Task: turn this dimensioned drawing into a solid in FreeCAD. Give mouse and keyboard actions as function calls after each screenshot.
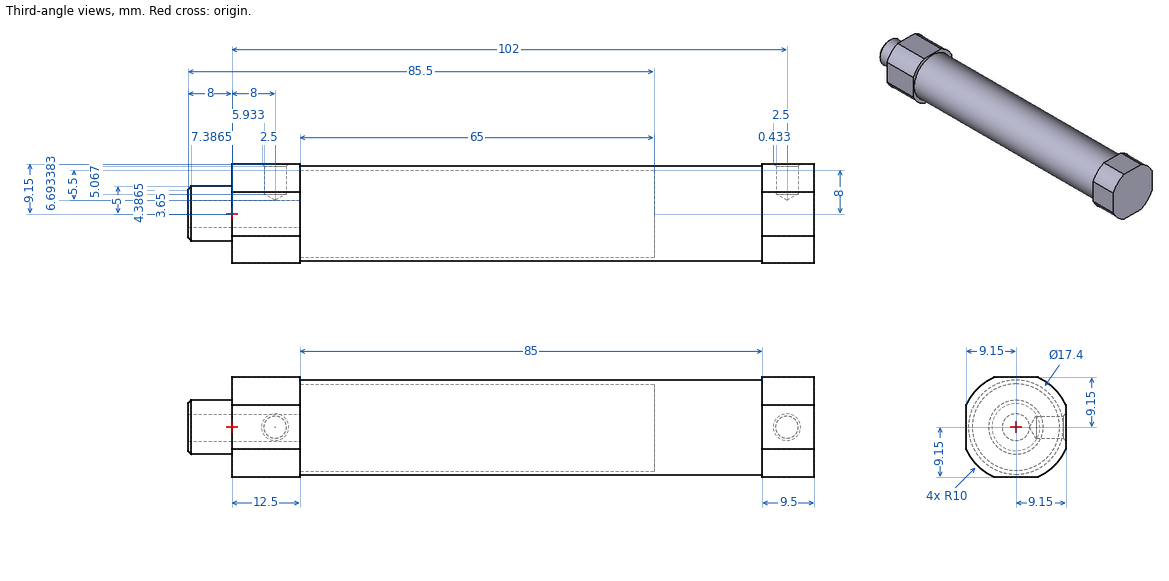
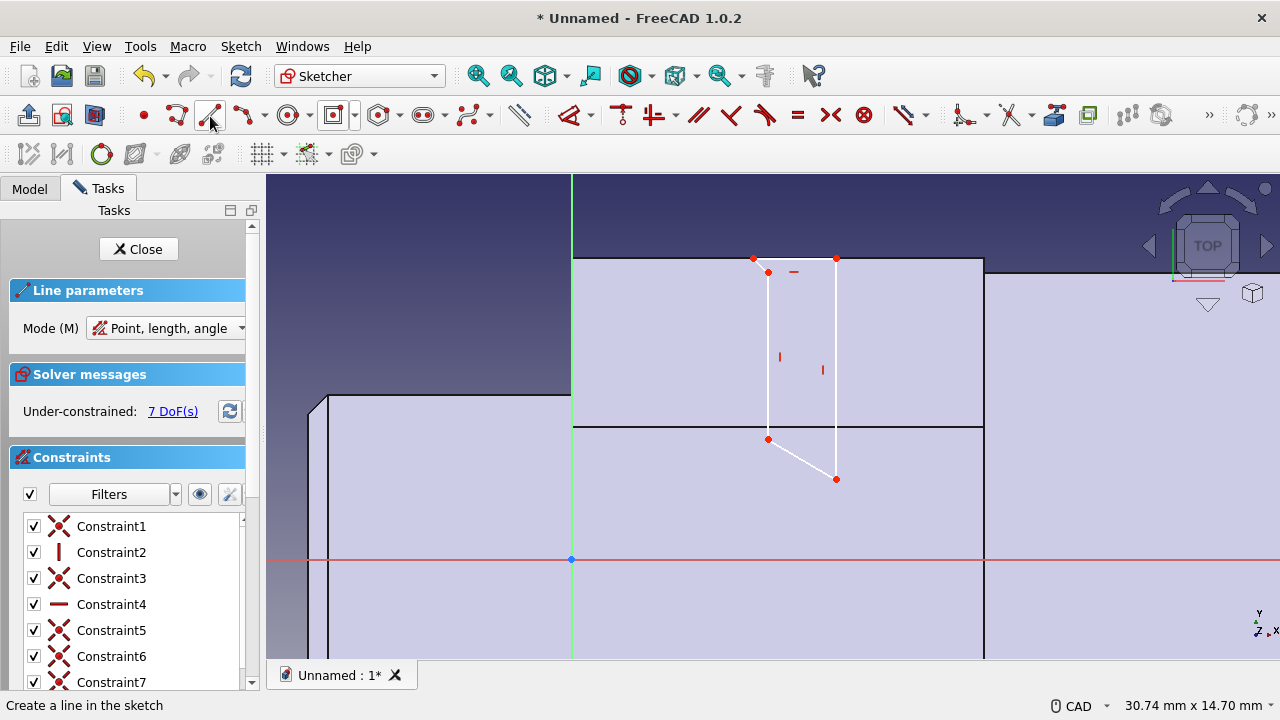
click(836, 501)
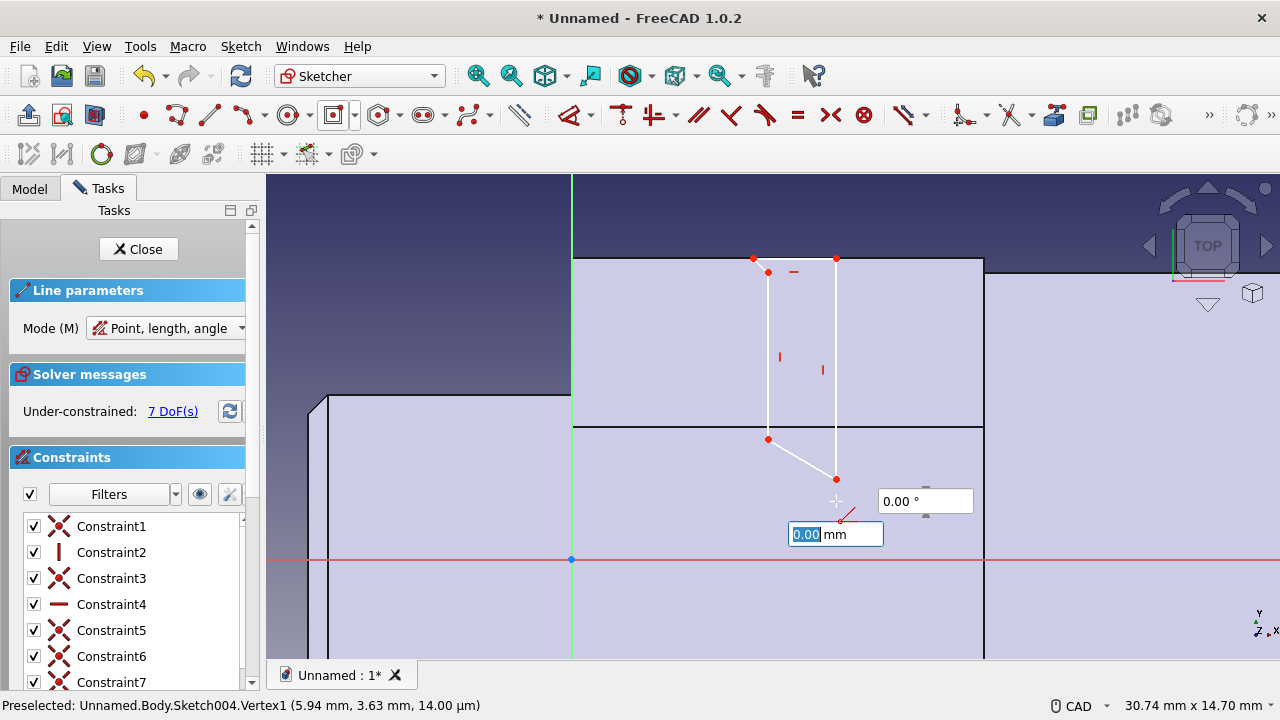
scroll(836, 567, up, 4)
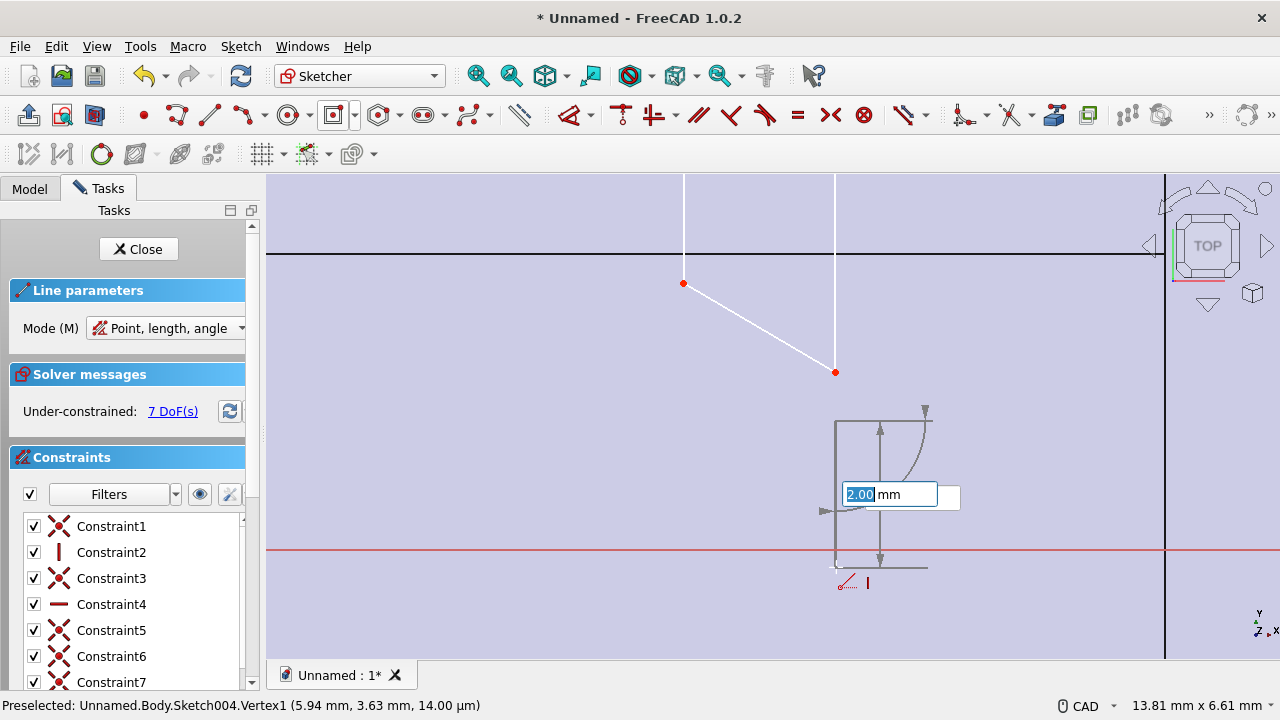
click(835, 566)
key(Escape)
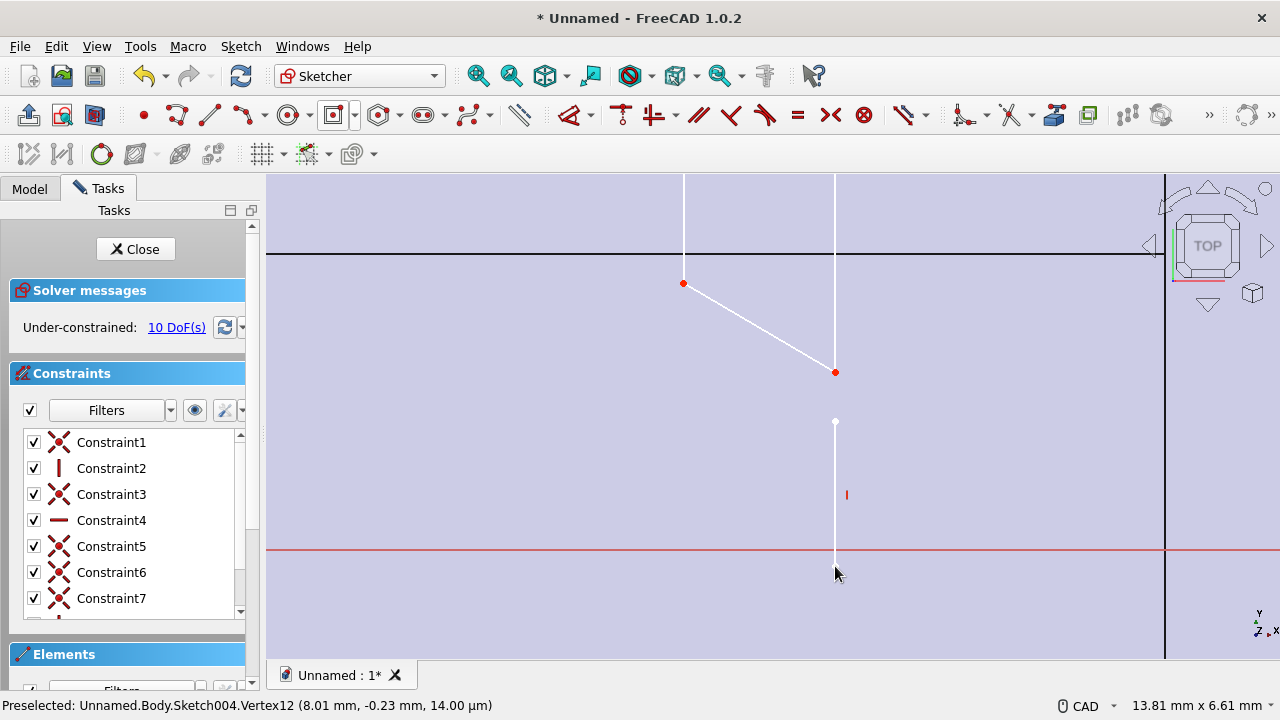
click(835, 465)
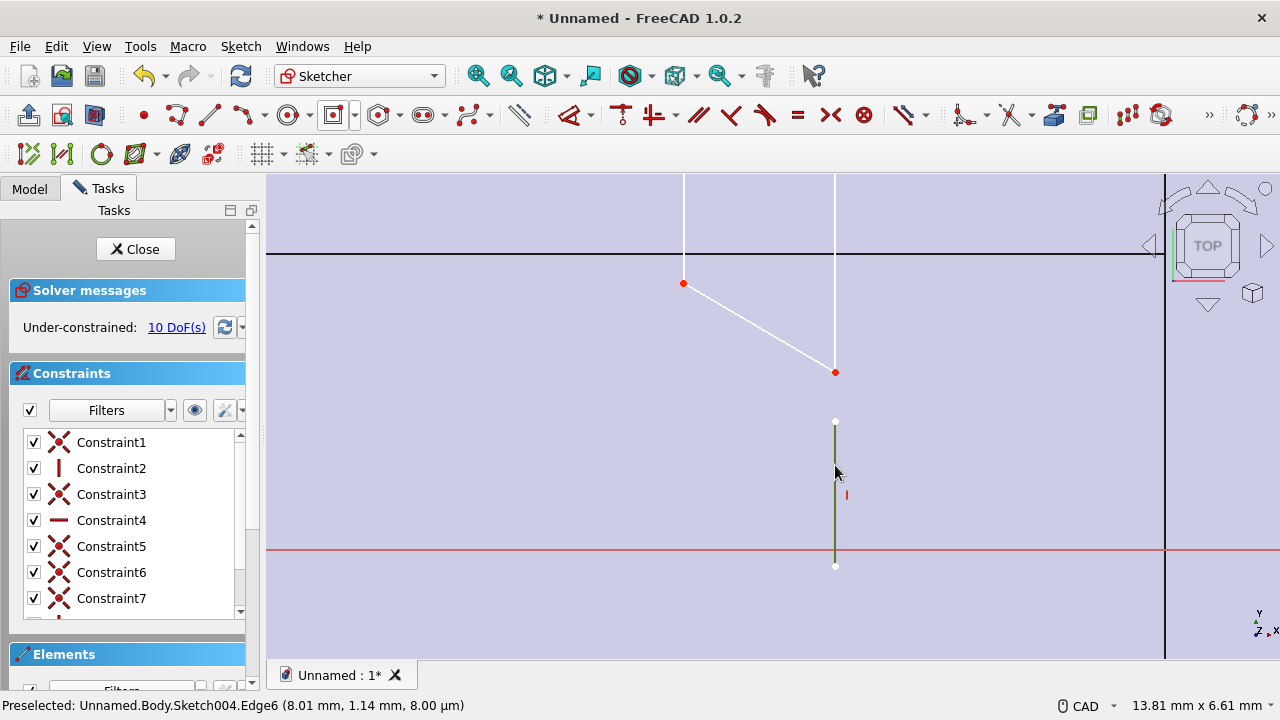
click(520, 116)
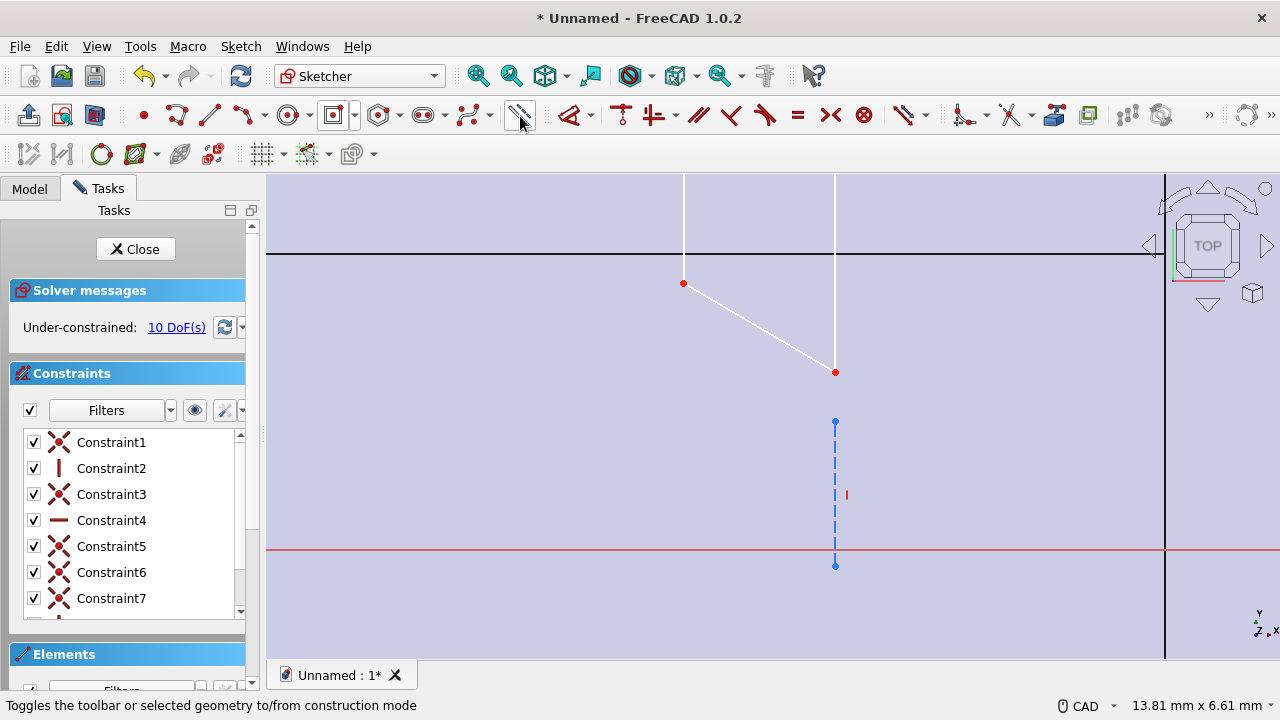
click(568, 116)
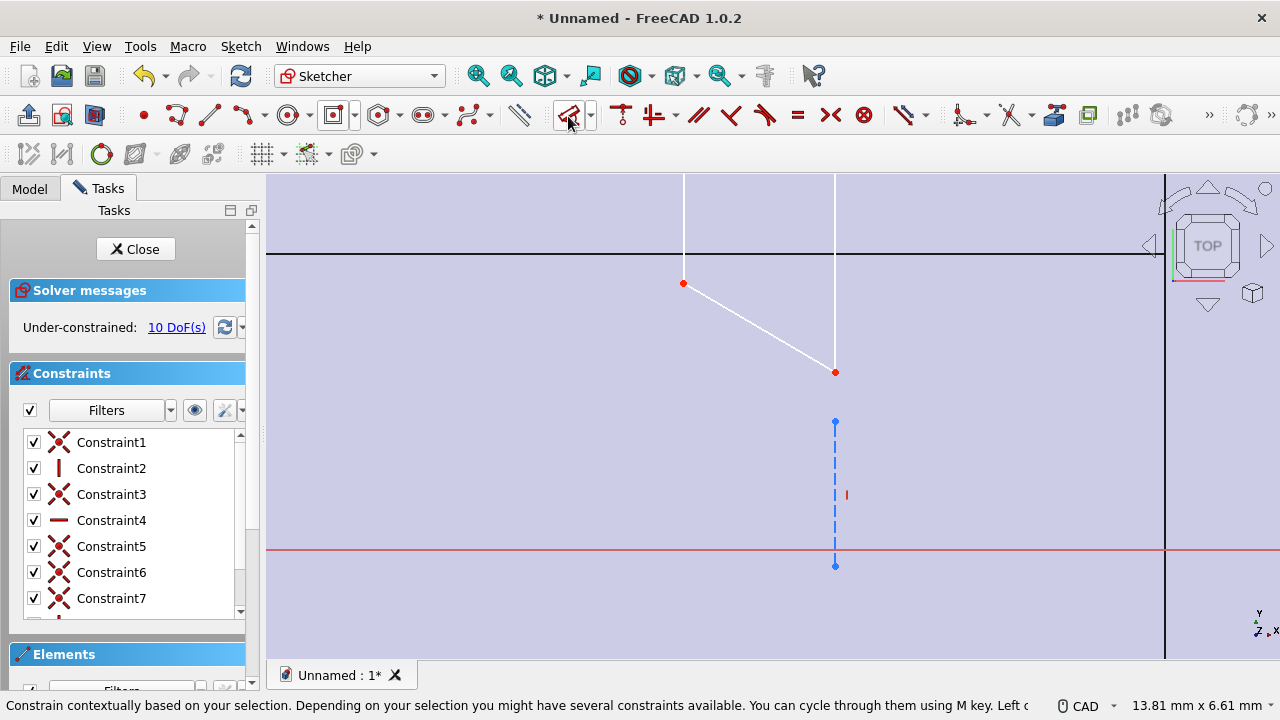
click(835, 372)
click(565, 584)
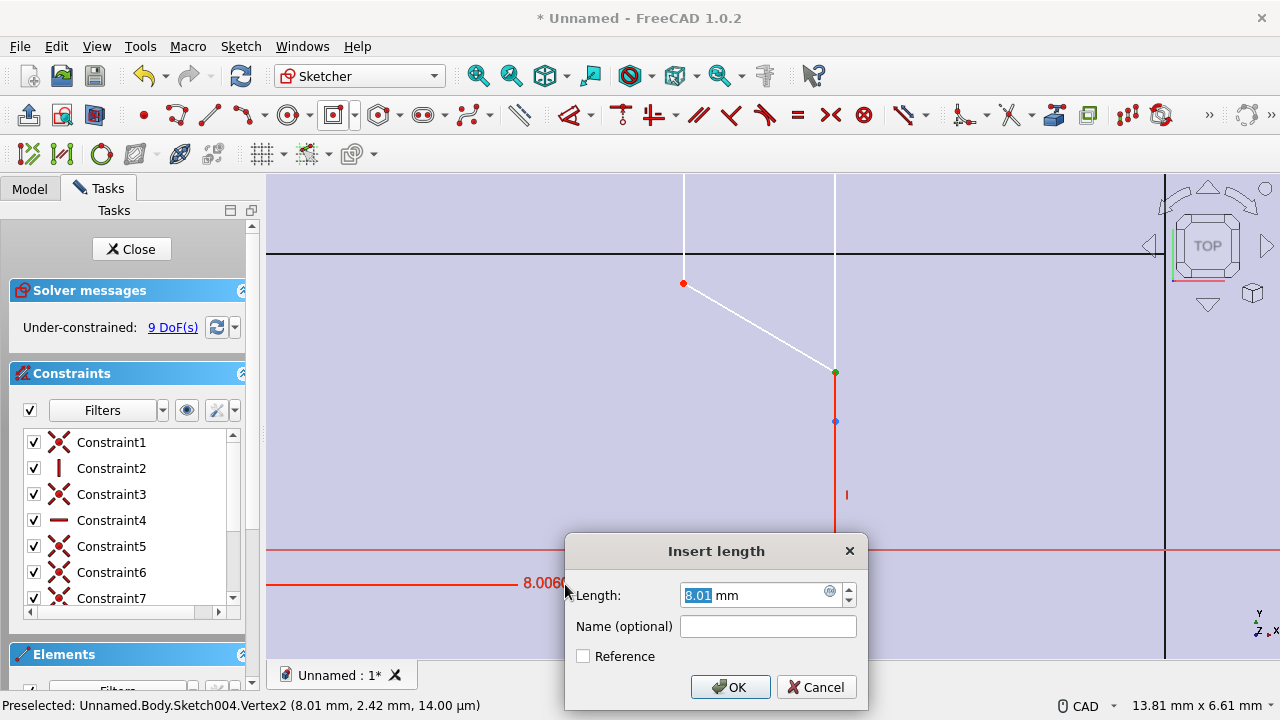
text(8)
key(Return)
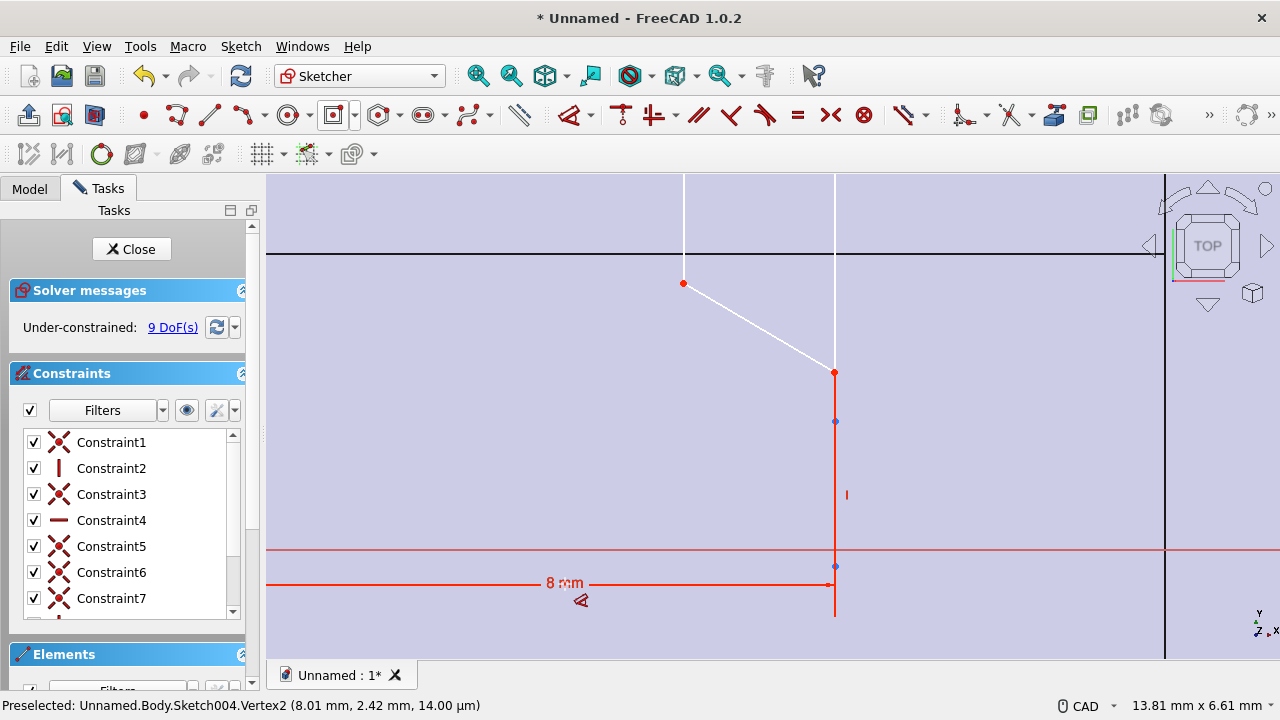
click(835, 421)
click(440, 584)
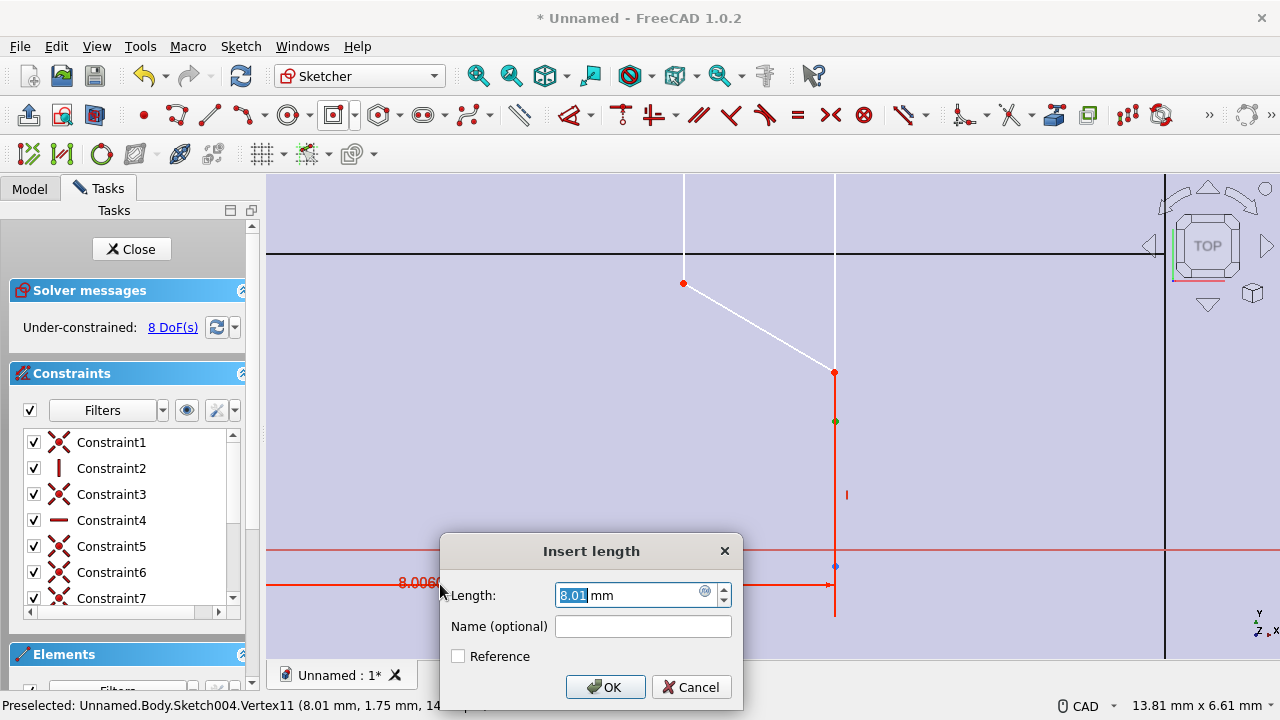
text(8)
key(Return)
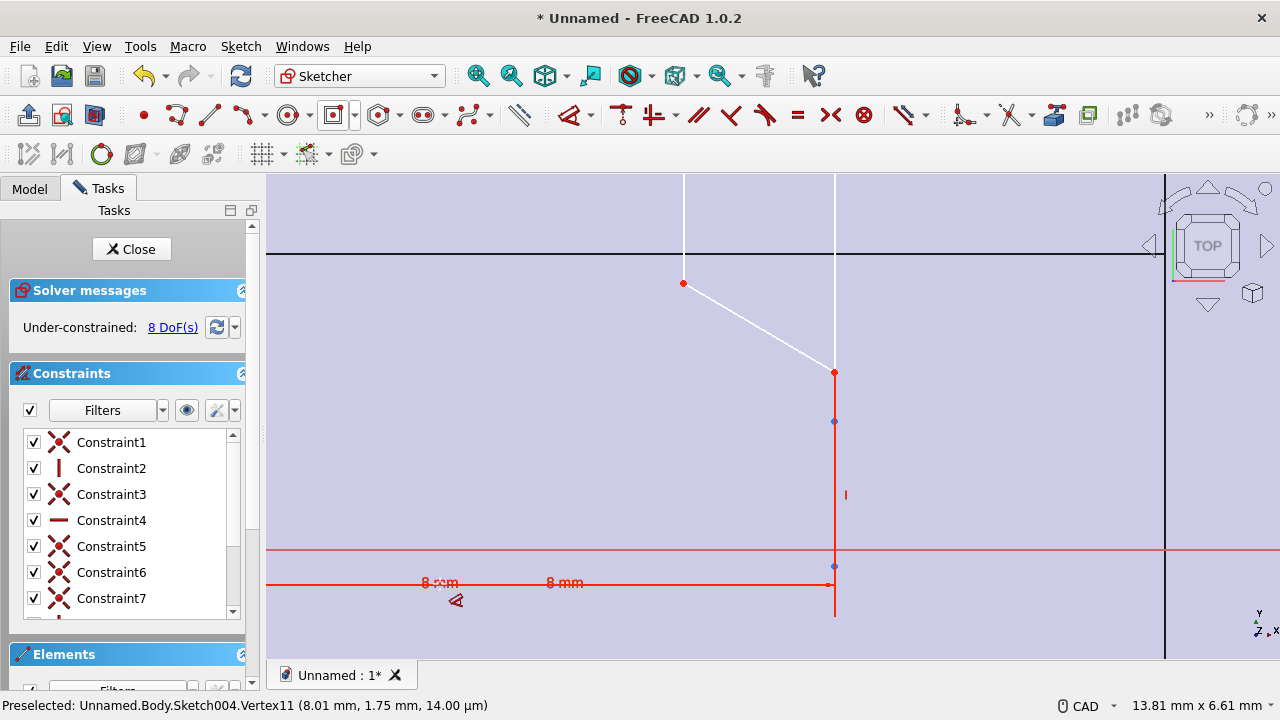
scroll(838, 575, down, 4)